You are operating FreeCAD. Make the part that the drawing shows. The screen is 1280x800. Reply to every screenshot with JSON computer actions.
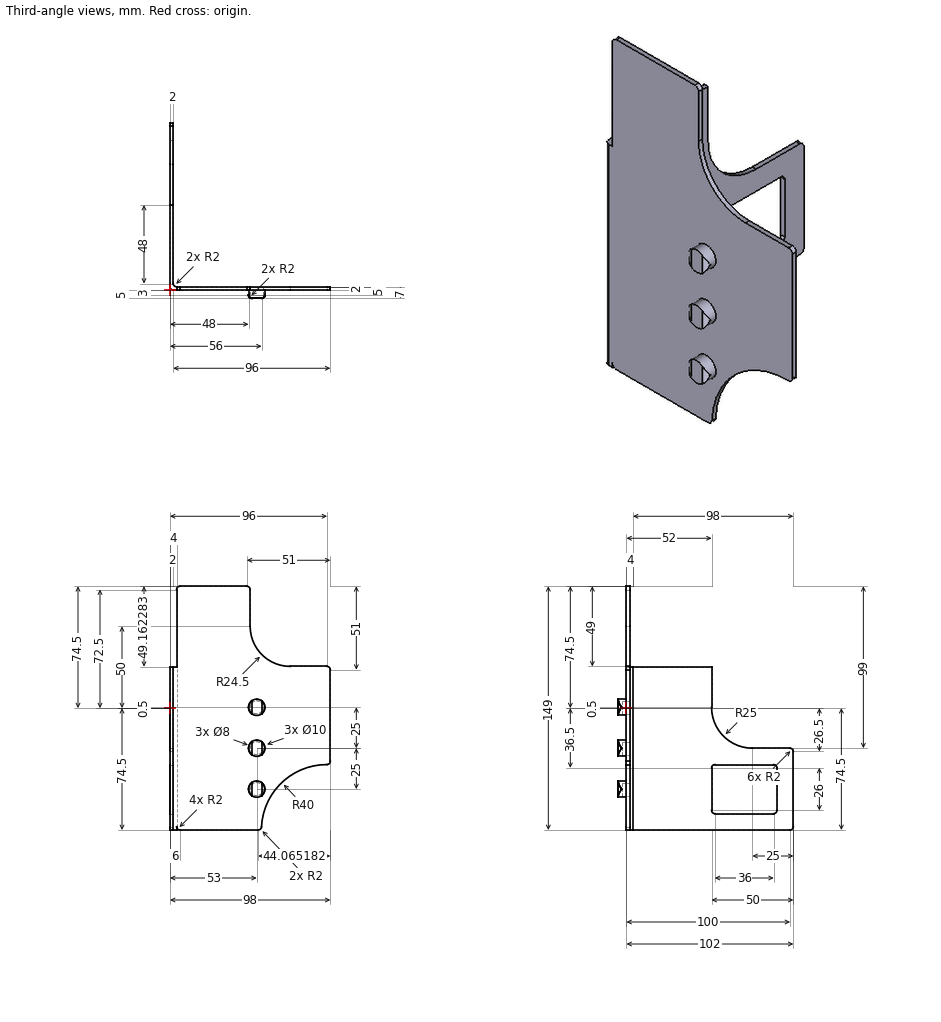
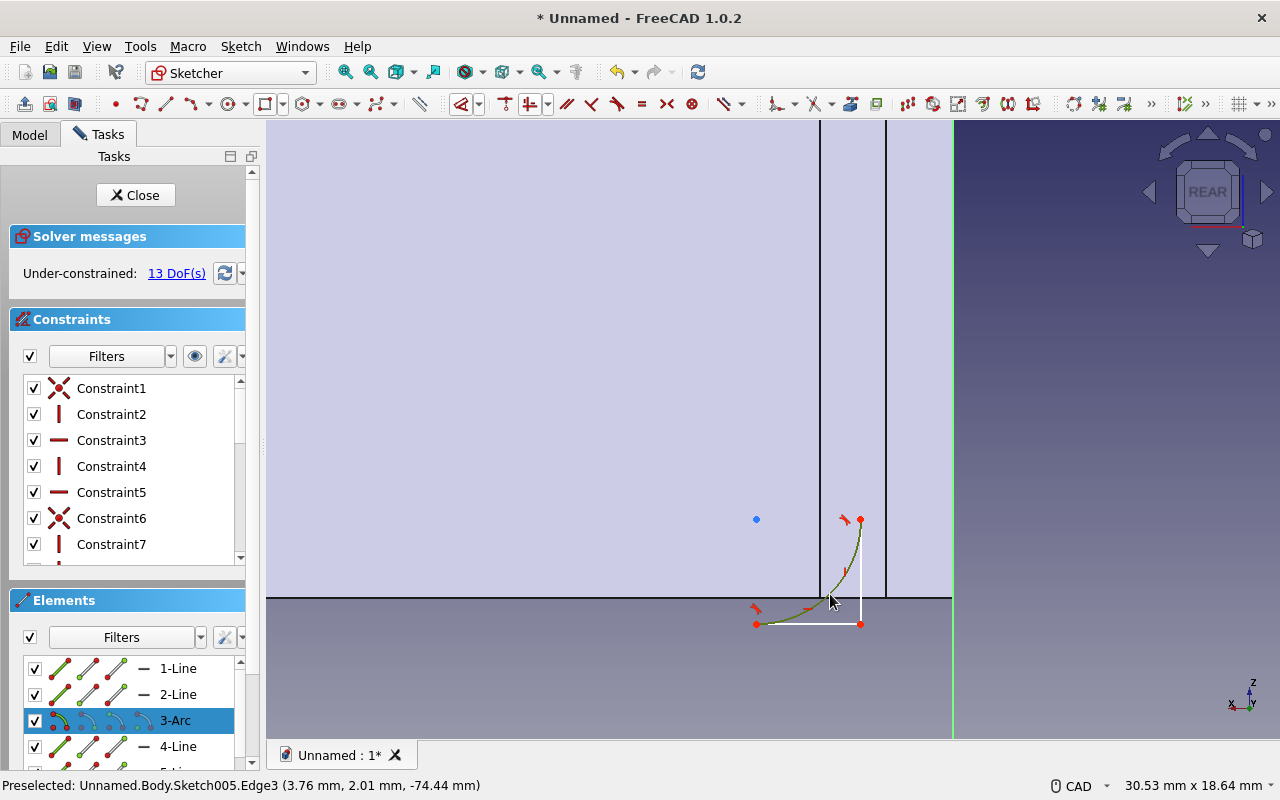
{"action": "scroll", "coordinate": [815, 615], "scroll_direction": "down", "scroll_amount": 13}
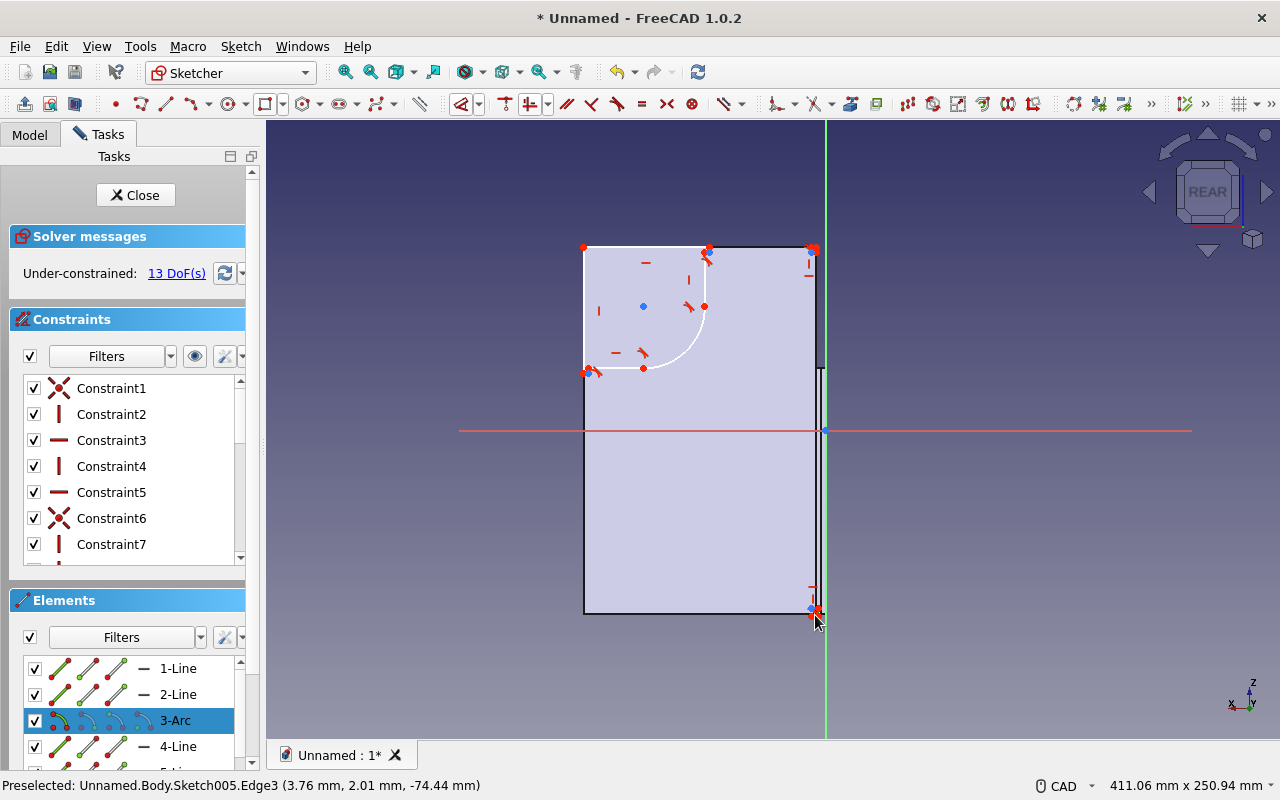
{"action": "scroll", "coordinate": [705, 250], "scroll_direction": "up", "scroll_amount": 9}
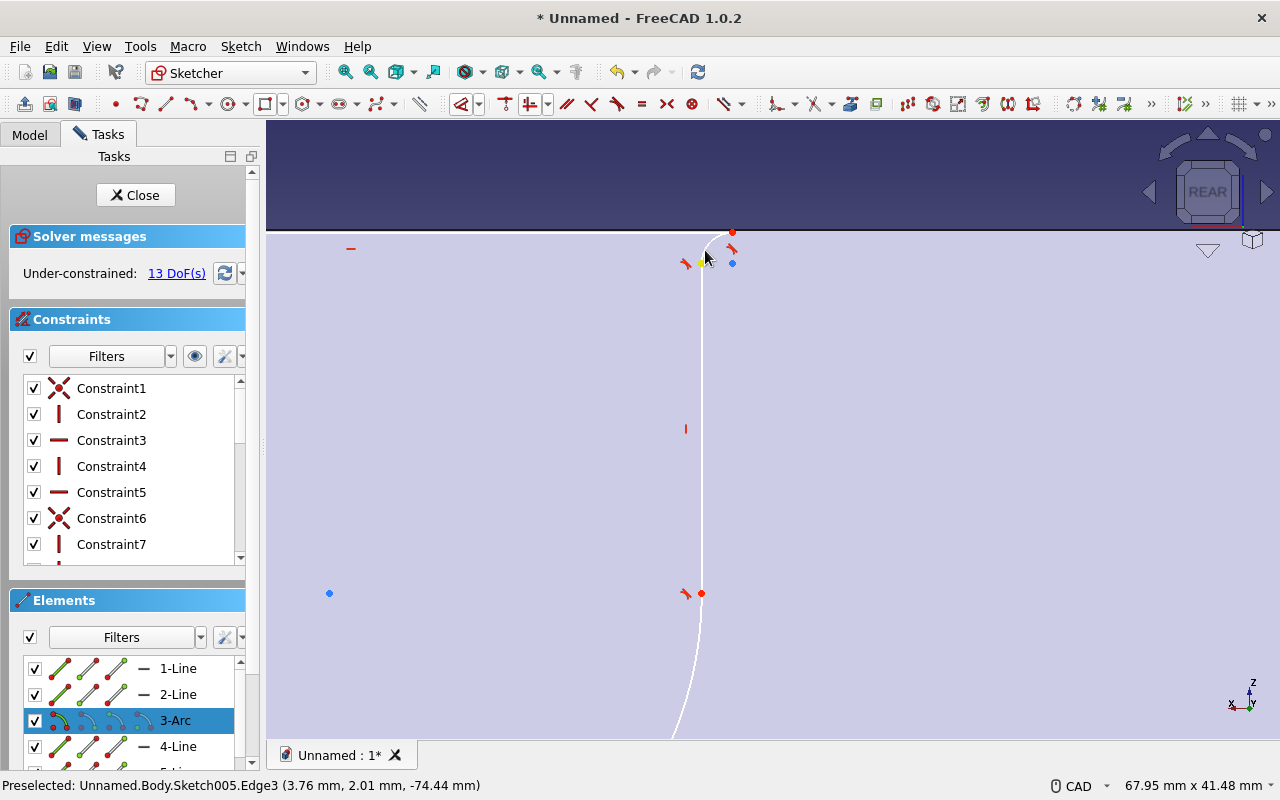
{"action": "left_click", "coordinate": [705, 250]}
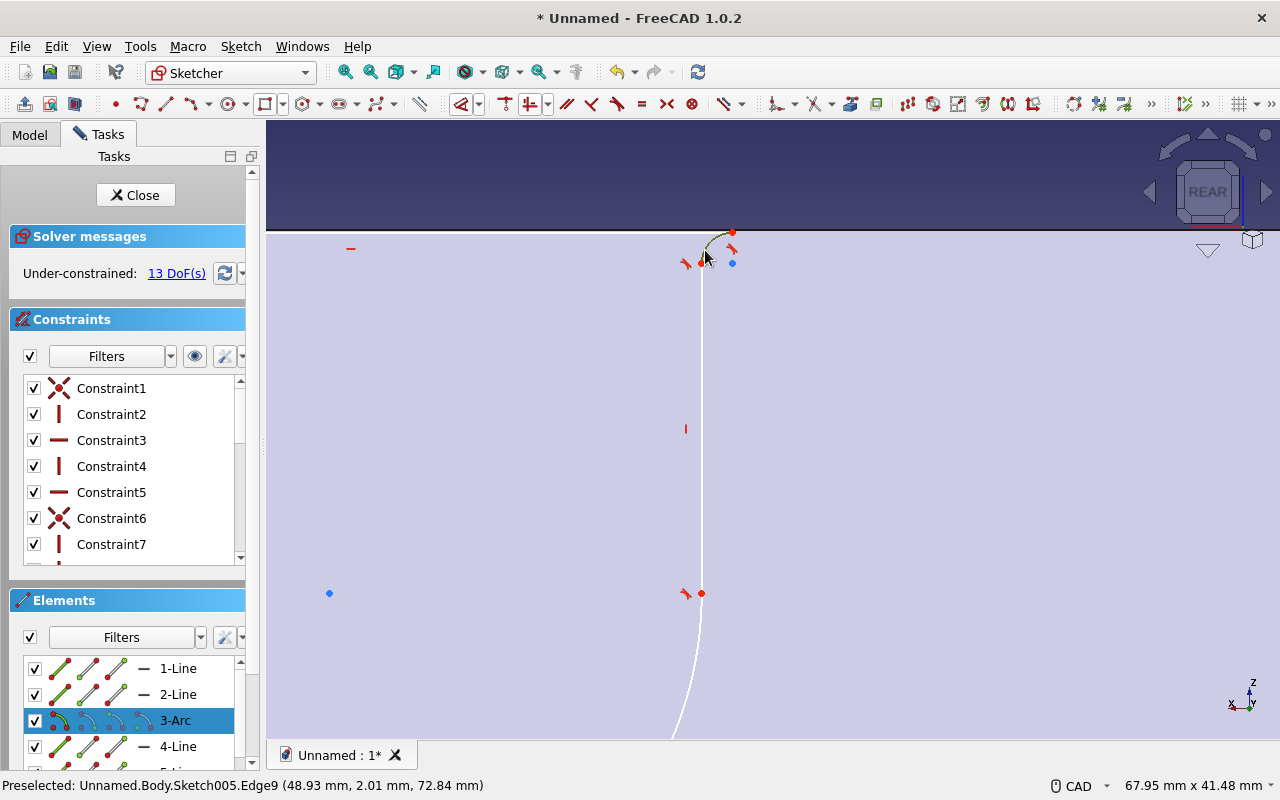
{"action": "scroll", "coordinate": [705, 249], "scroll_direction": "down", "scroll_amount": 9}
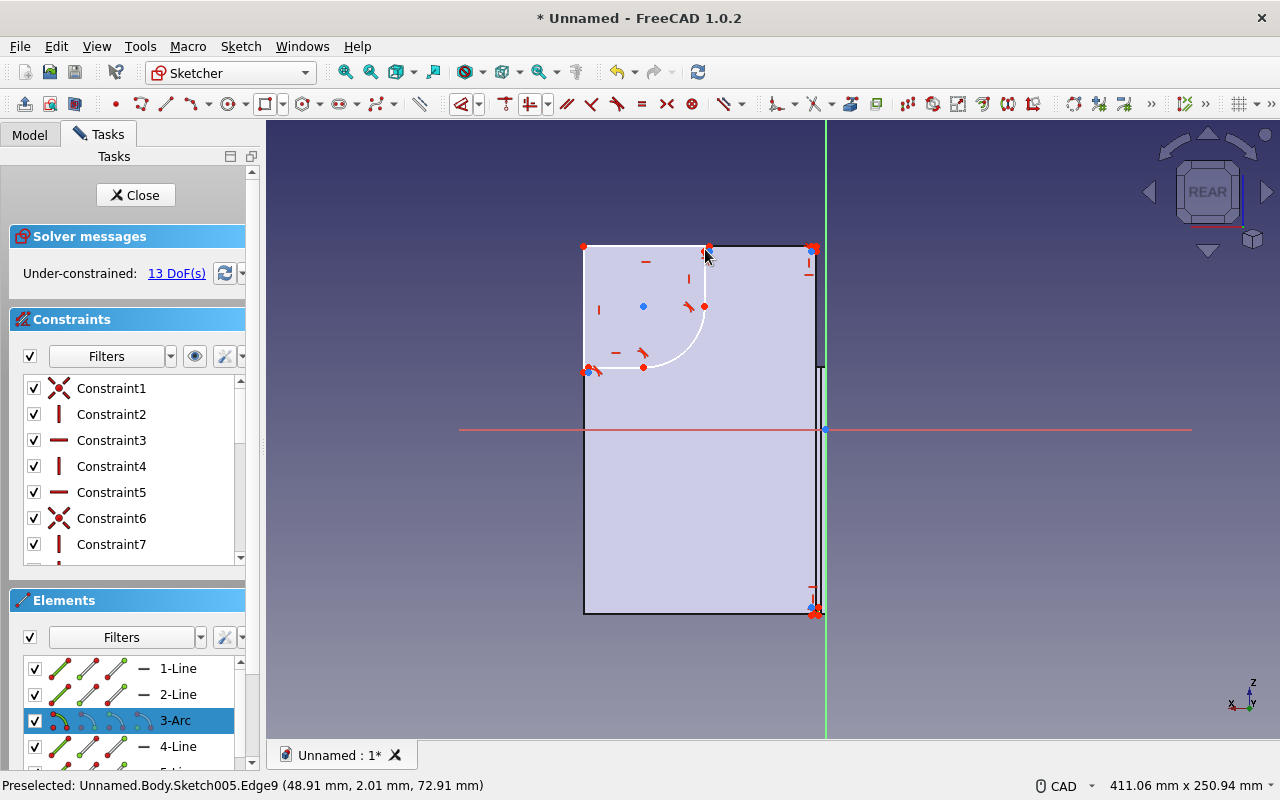
{"action": "scroll", "coordinate": [587, 368], "scroll_direction": "up", "scroll_amount": 10}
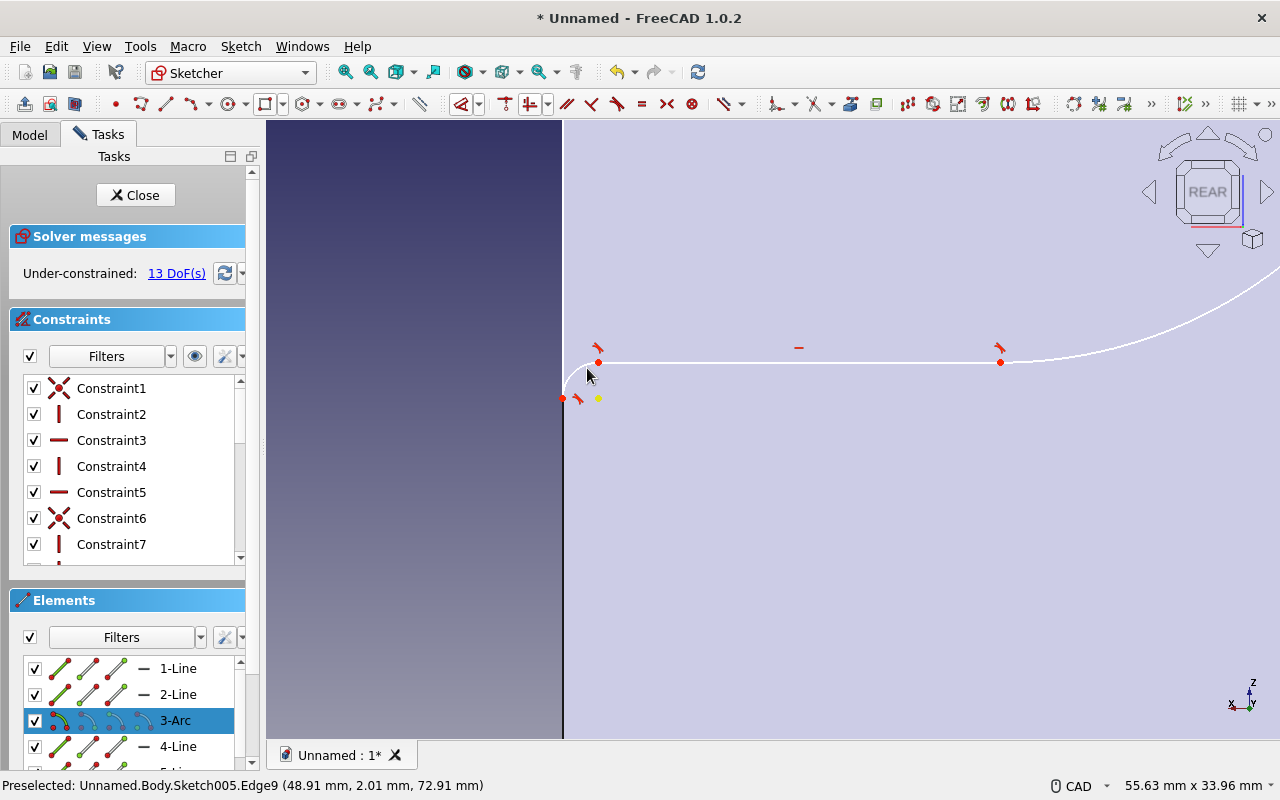
{"action": "left_click", "coordinate": [582, 367]}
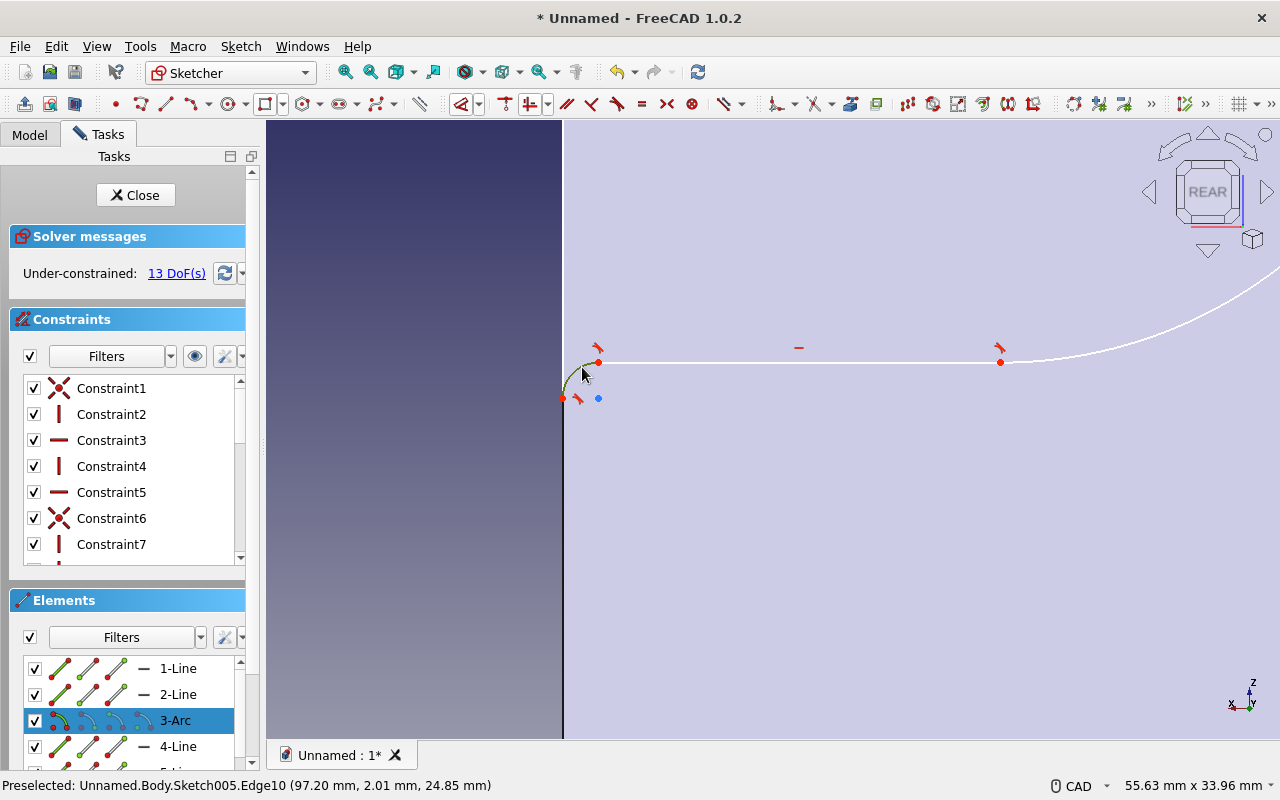
{"action": "scroll", "coordinate": [587, 368], "scroll_direction": "down", "scroll_amount": 10}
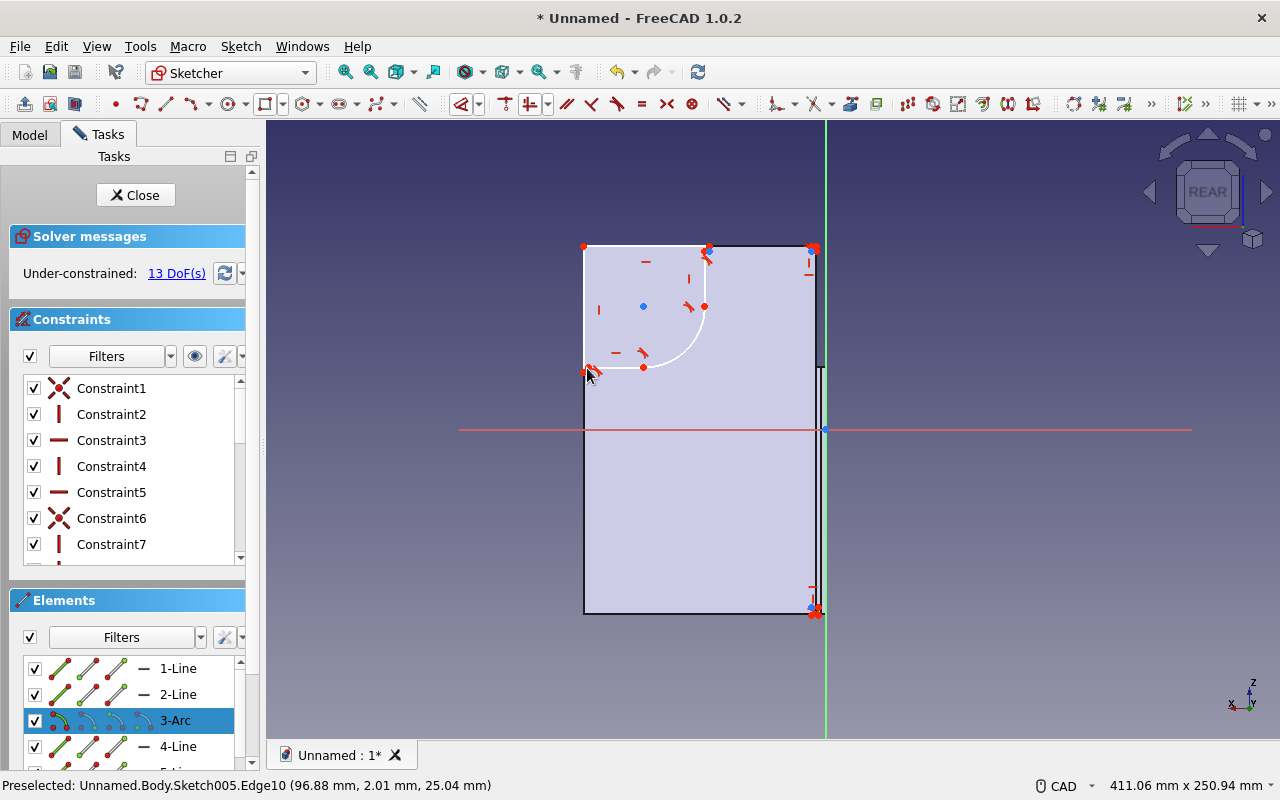
{"action": "scroll", "coordinate": [815, 248], "scroll_direction": "up", "scroll_amount": 12}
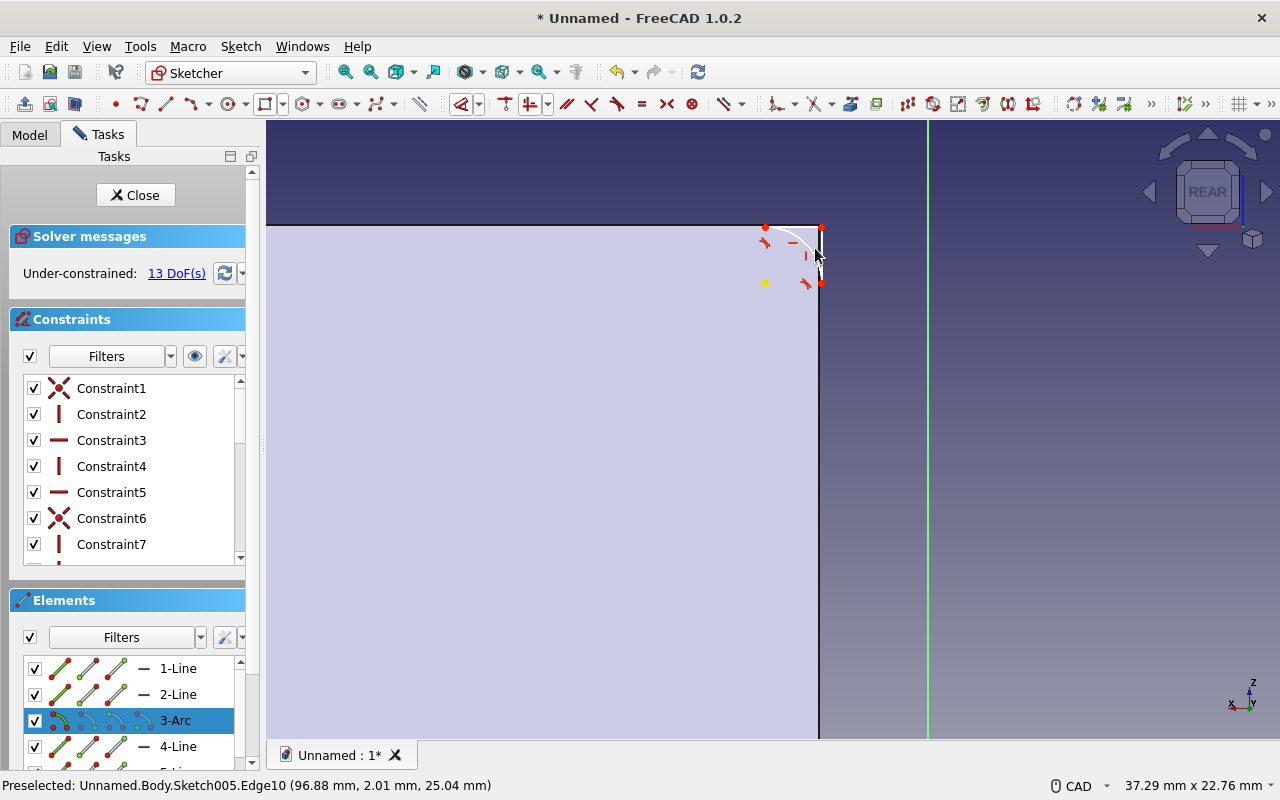
{"action": "left_click", "coordinate": [806, 244]}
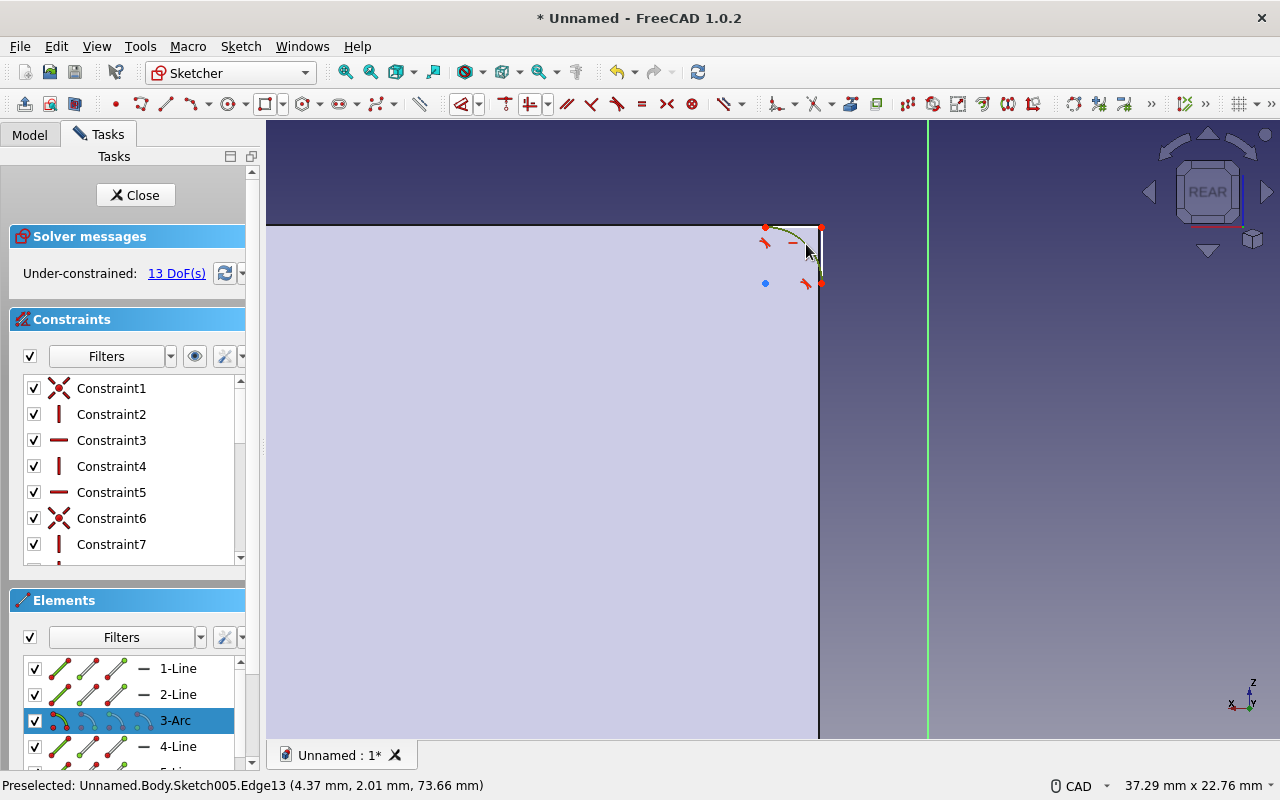
{"action": "left_click", "coordinate": [642, 104]}